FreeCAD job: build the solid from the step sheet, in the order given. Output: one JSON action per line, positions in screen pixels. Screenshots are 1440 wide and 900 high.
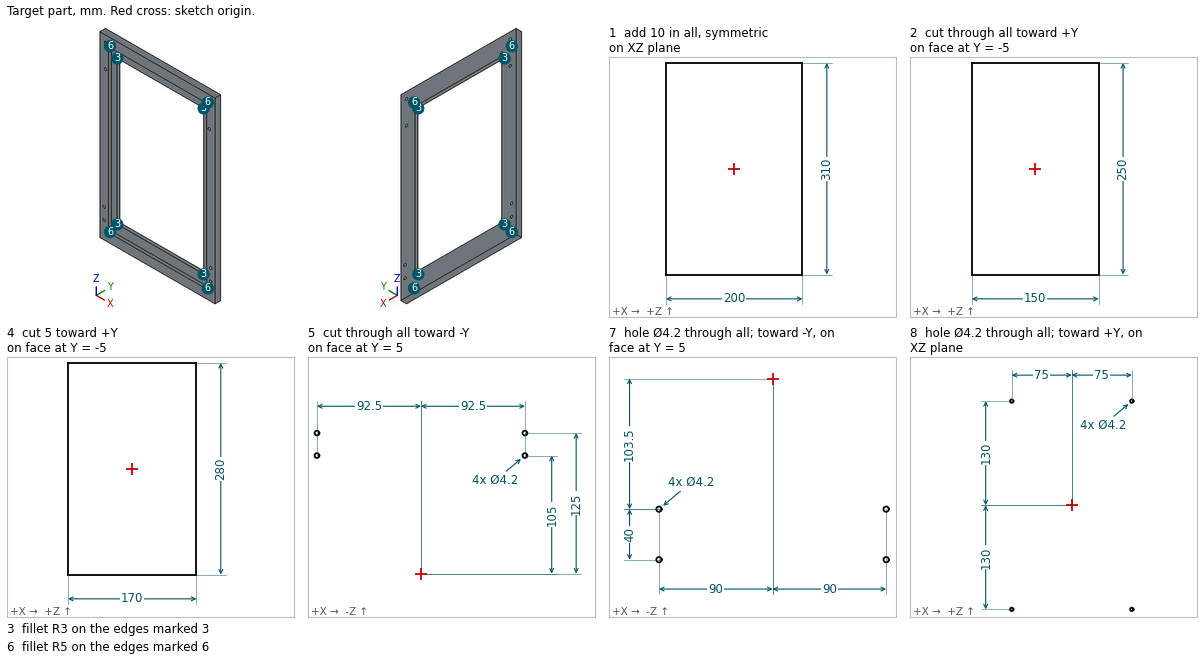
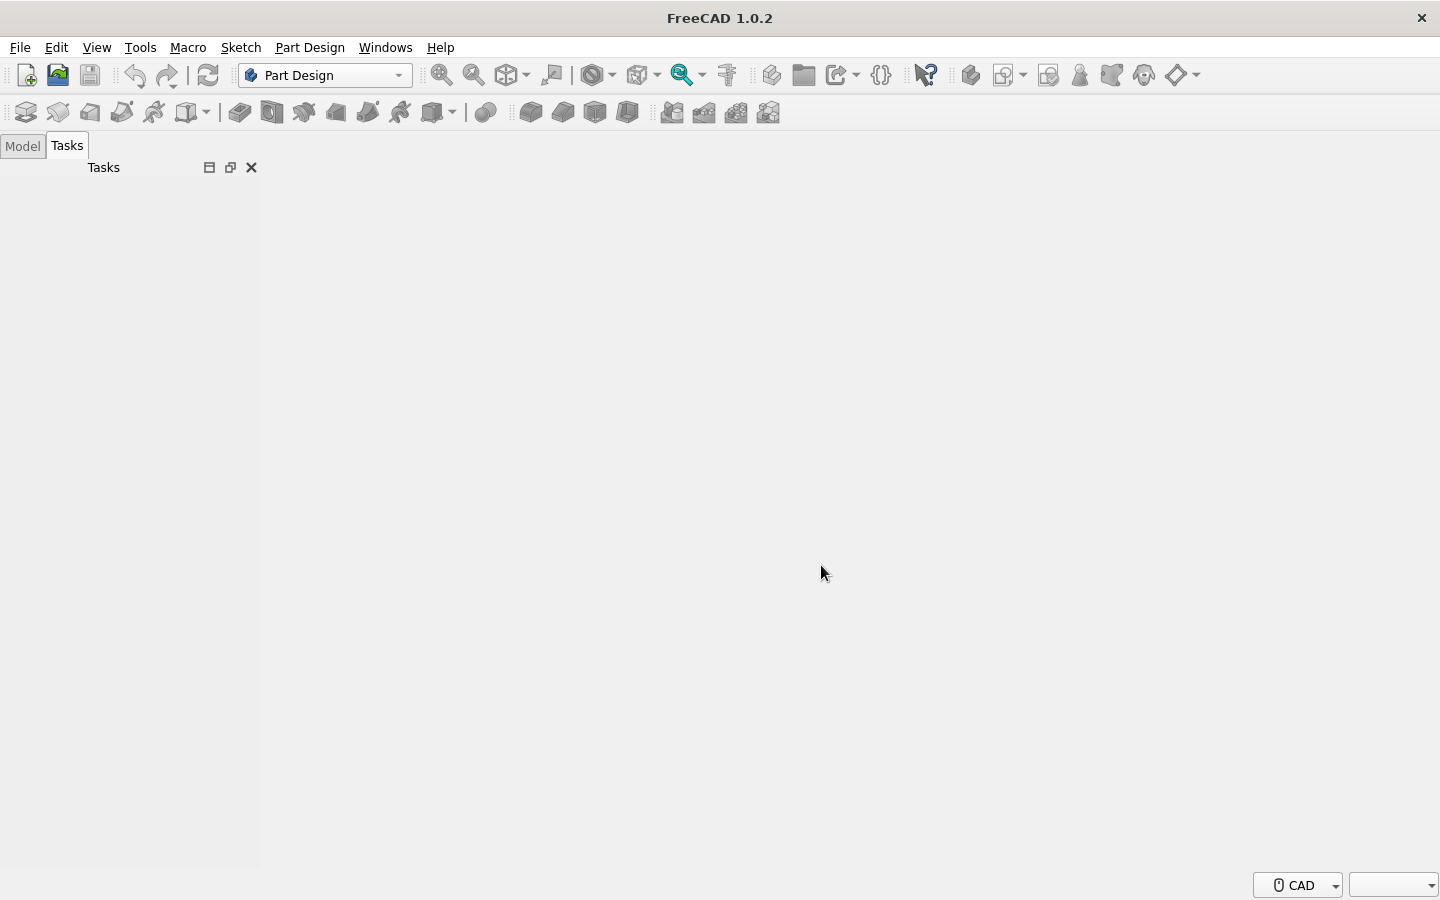
{"action": "key", "text": "ctrl+n"}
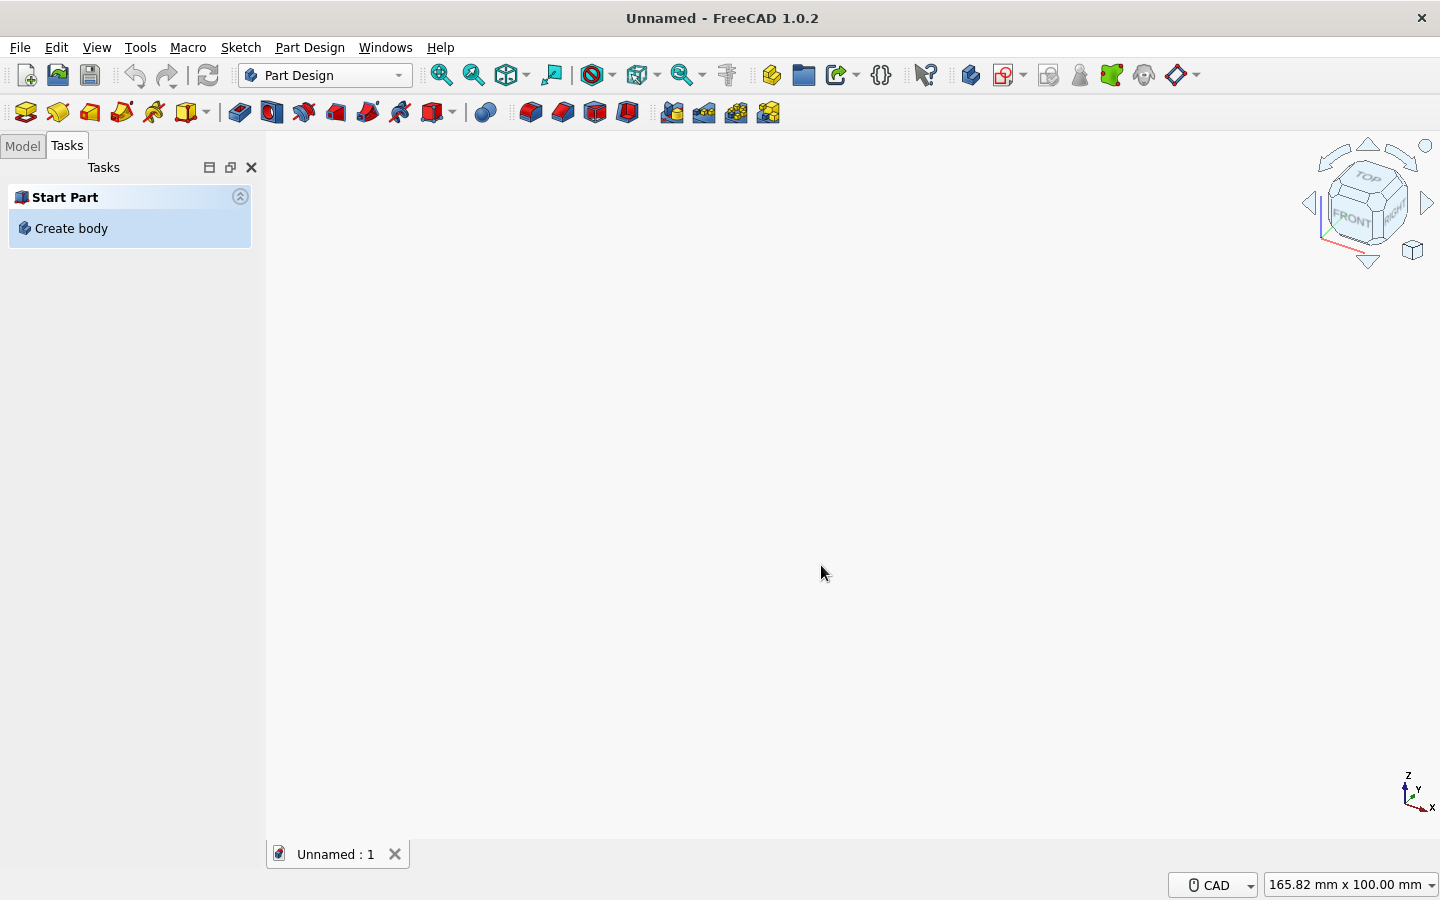
{"action": "left_click", "coordinate": [1004, 76]}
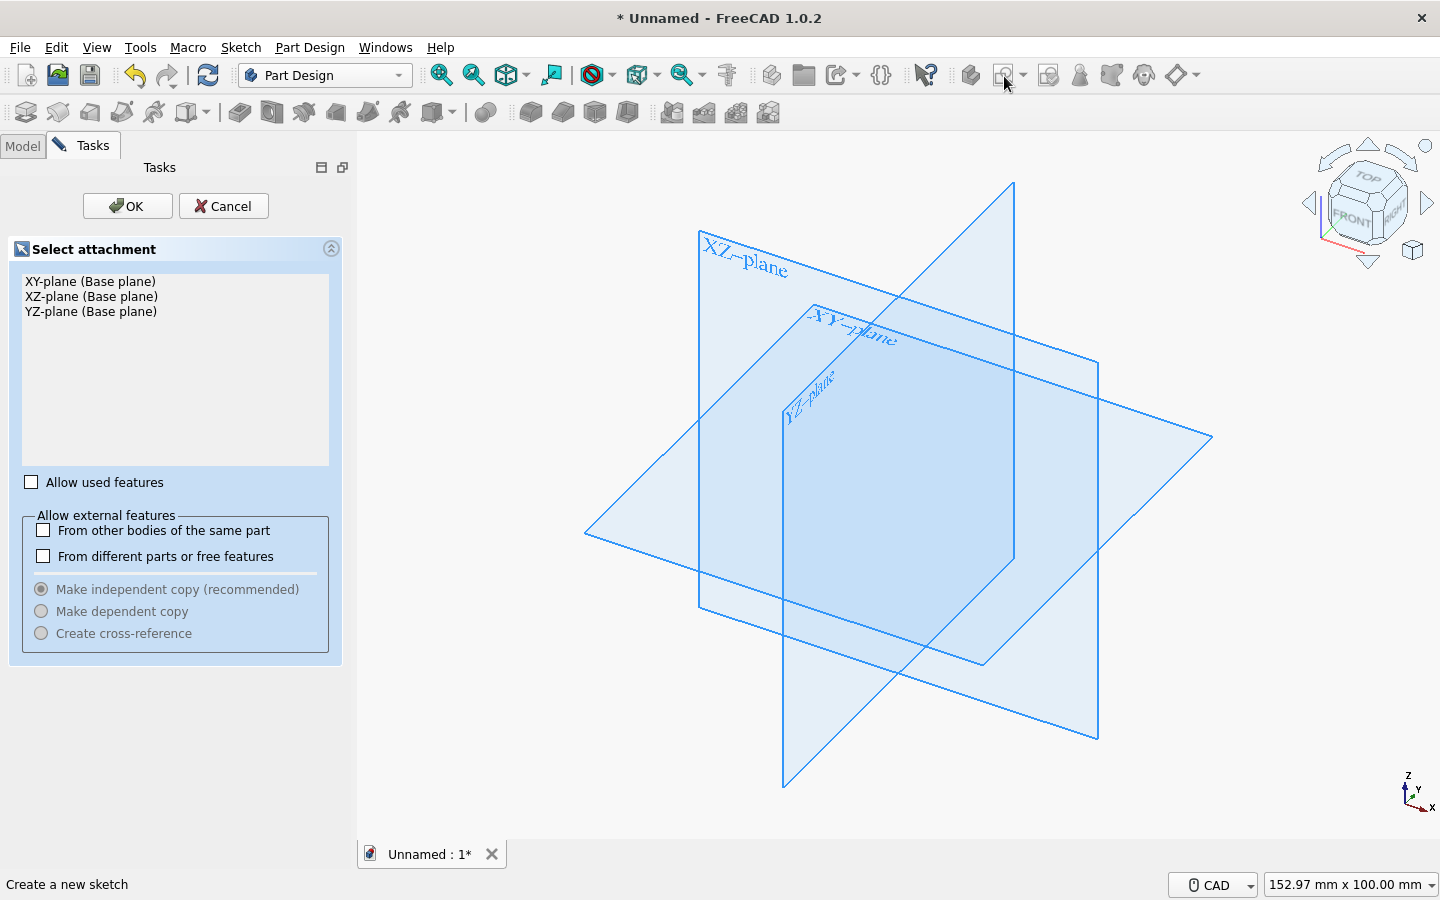
{"action": "left_click", "coordinate": [82, 296]}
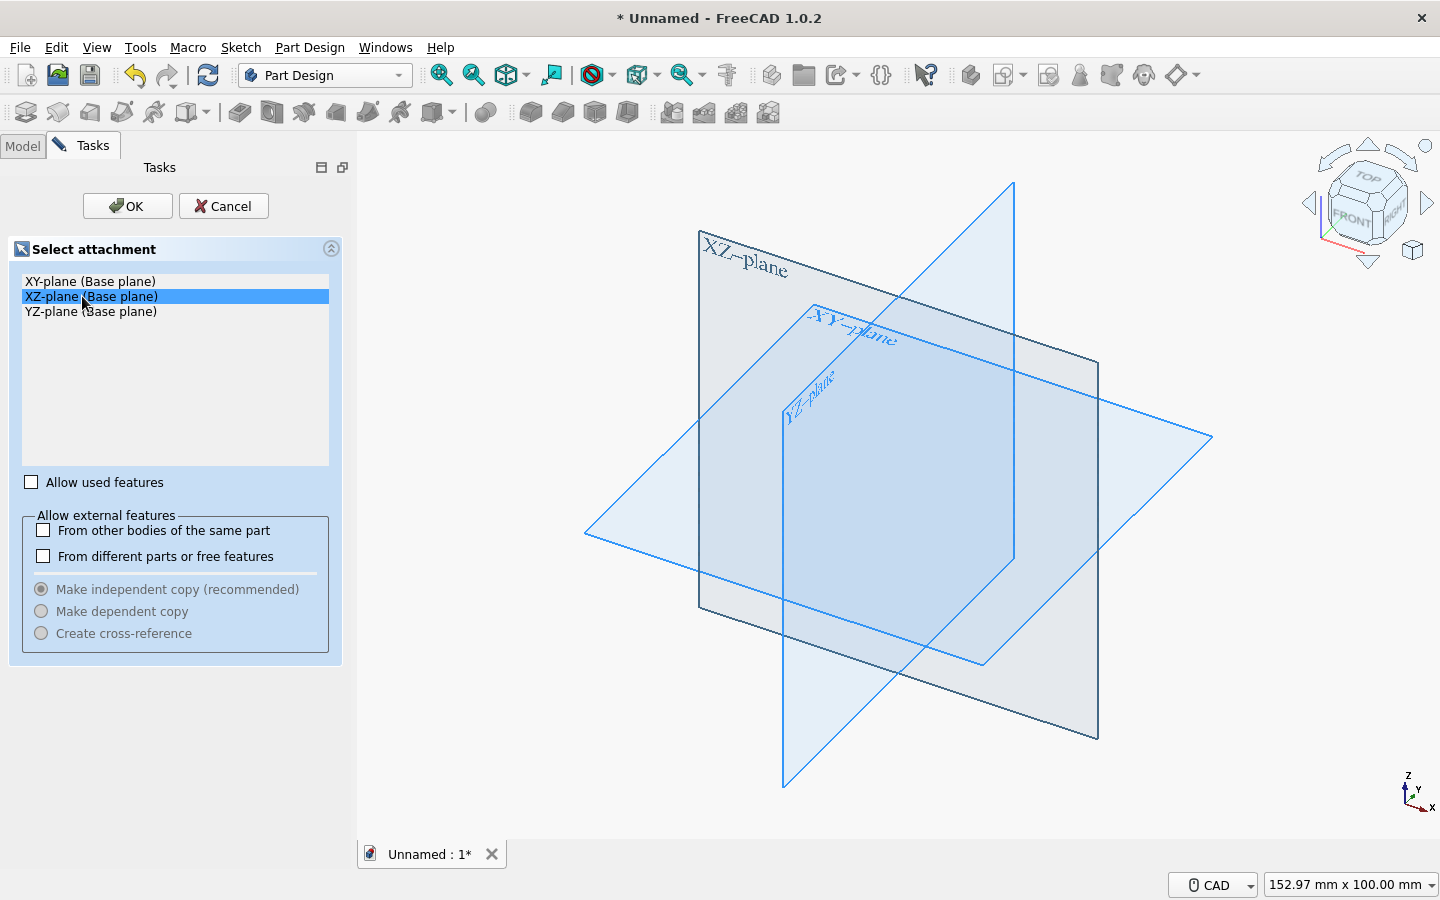
{"action": "left_click", "coordinate": [128, 206]}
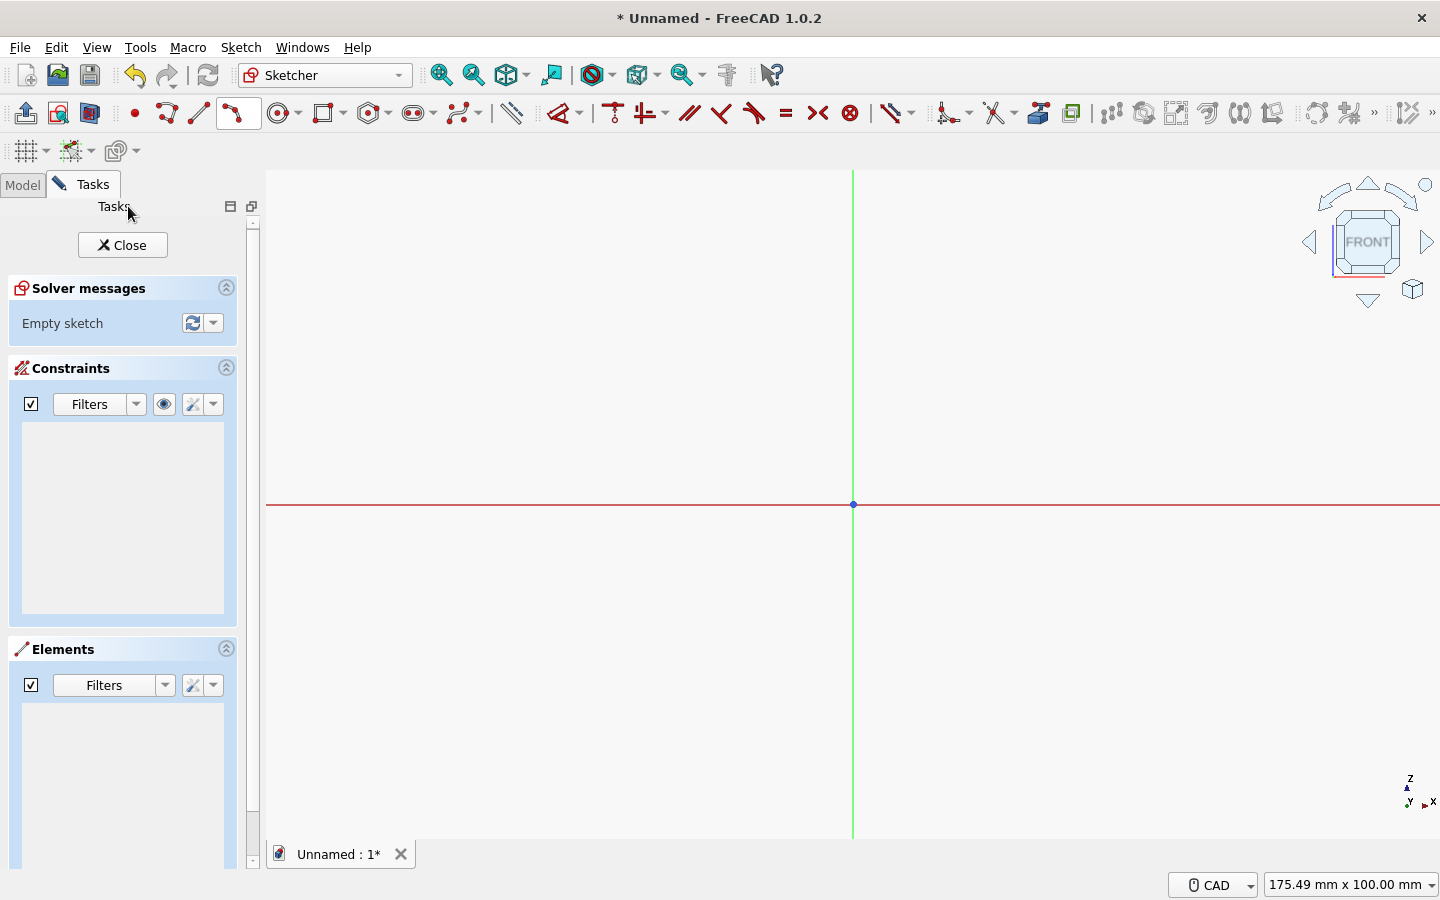
{"action": "scroll", "coordinate": [767, 504], "scroll_direction": "down", "scroll_amount": 8}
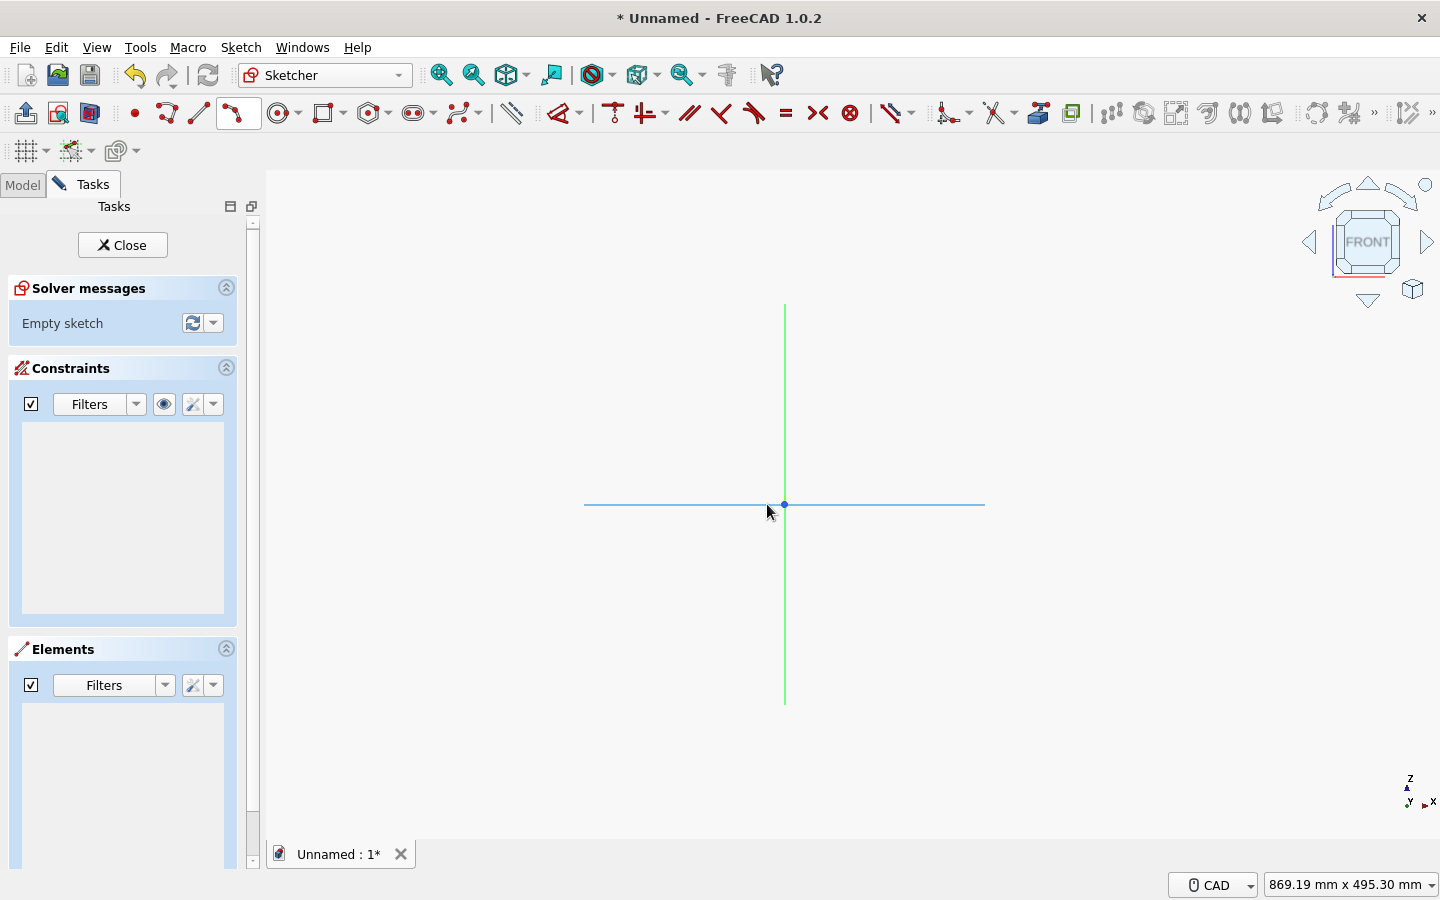
{"action": "key", "text": "g v"}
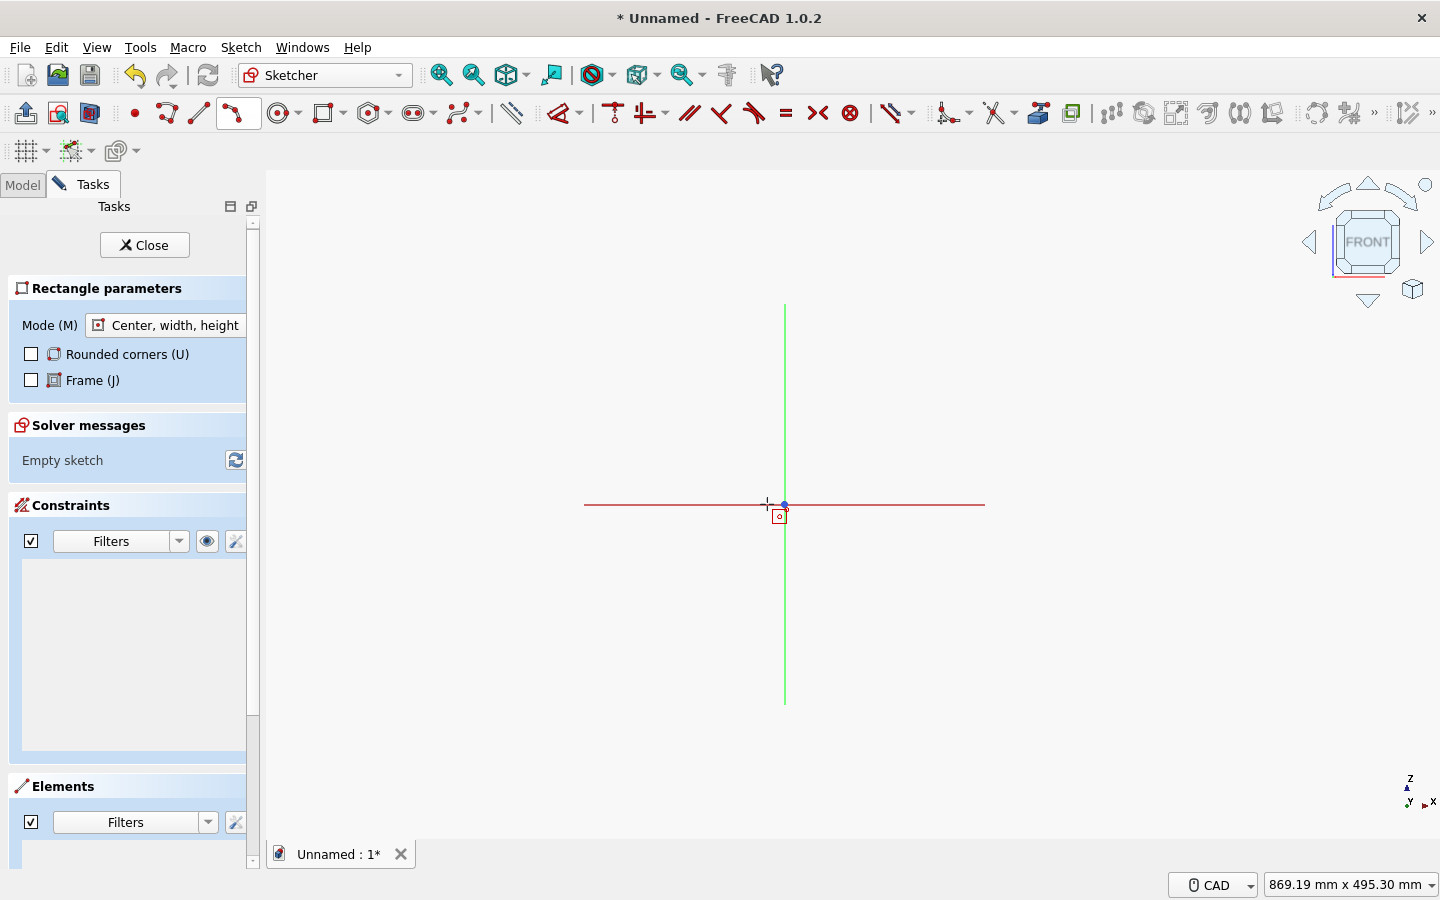
{"action": "left_click", "coordinate": [785, 504]}
{"action": "left_click", "coordinate": [920, 295]}
{"action": "key", "text": "Escape"}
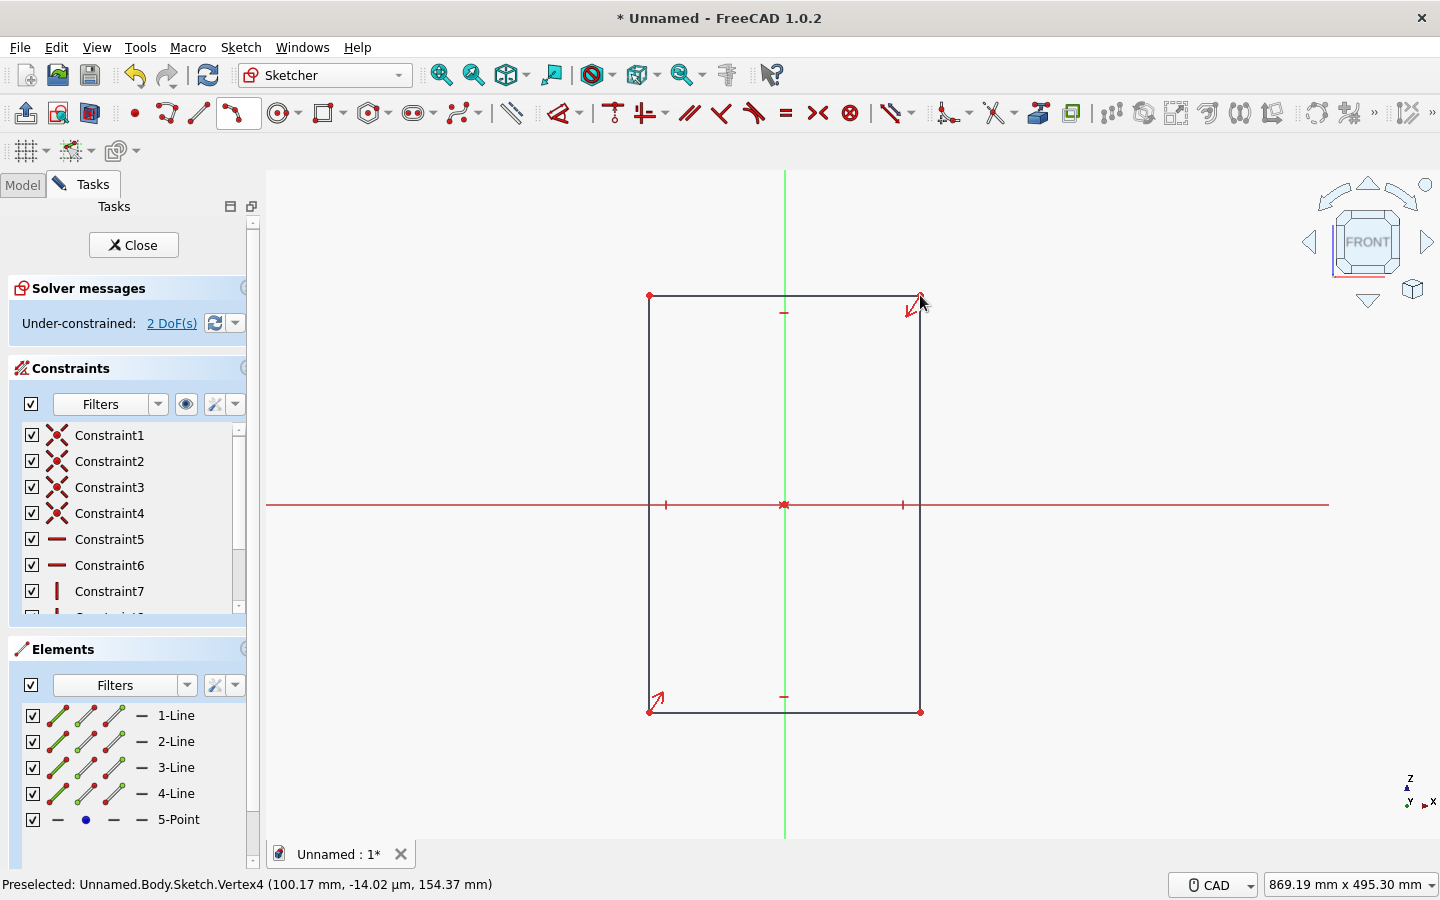
{"action": "left_click", "coordinate": [731, 713]}